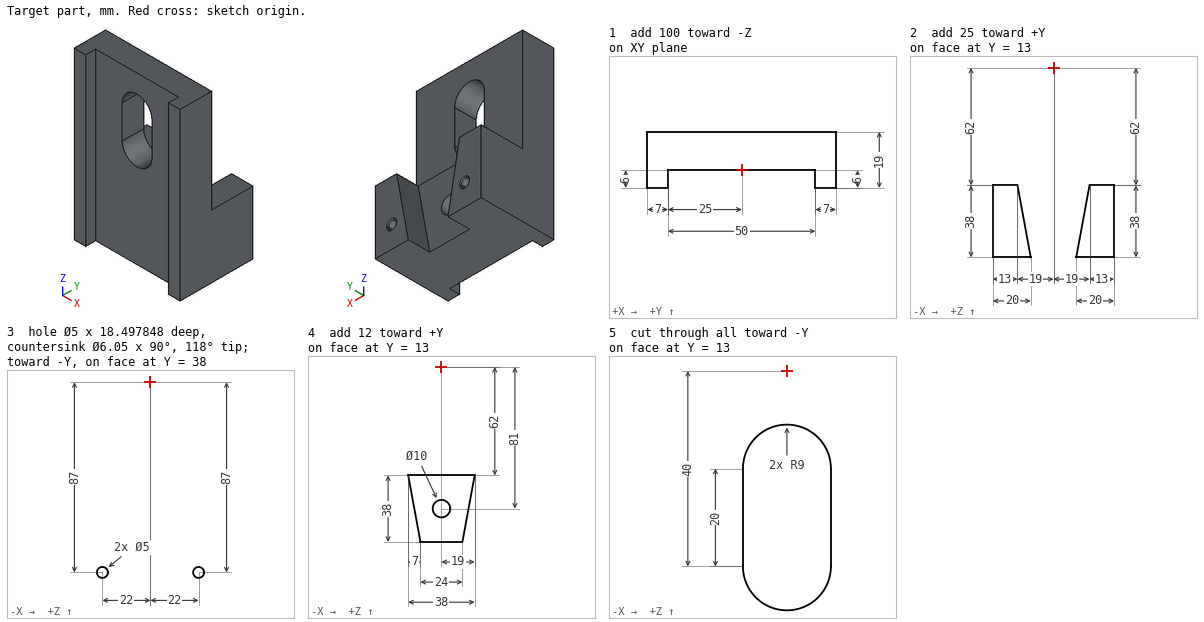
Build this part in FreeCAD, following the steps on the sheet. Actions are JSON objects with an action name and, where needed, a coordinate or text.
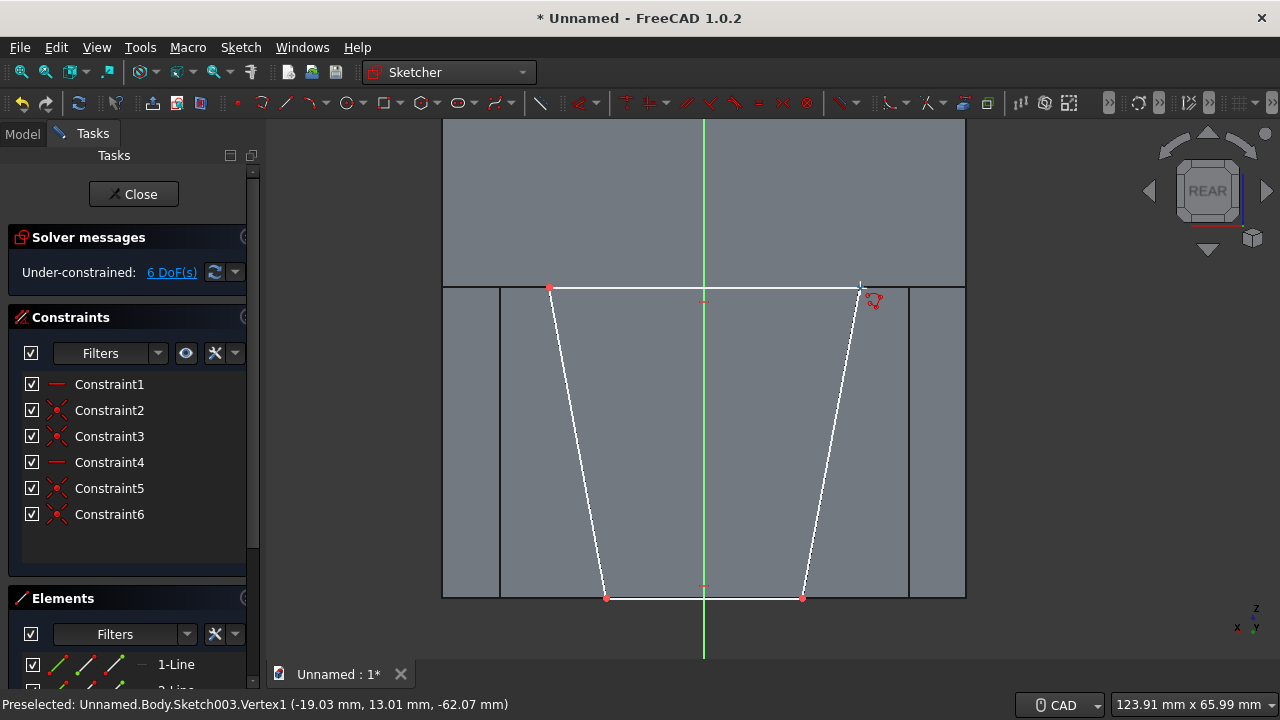
{"action": "key", "text": "g c"}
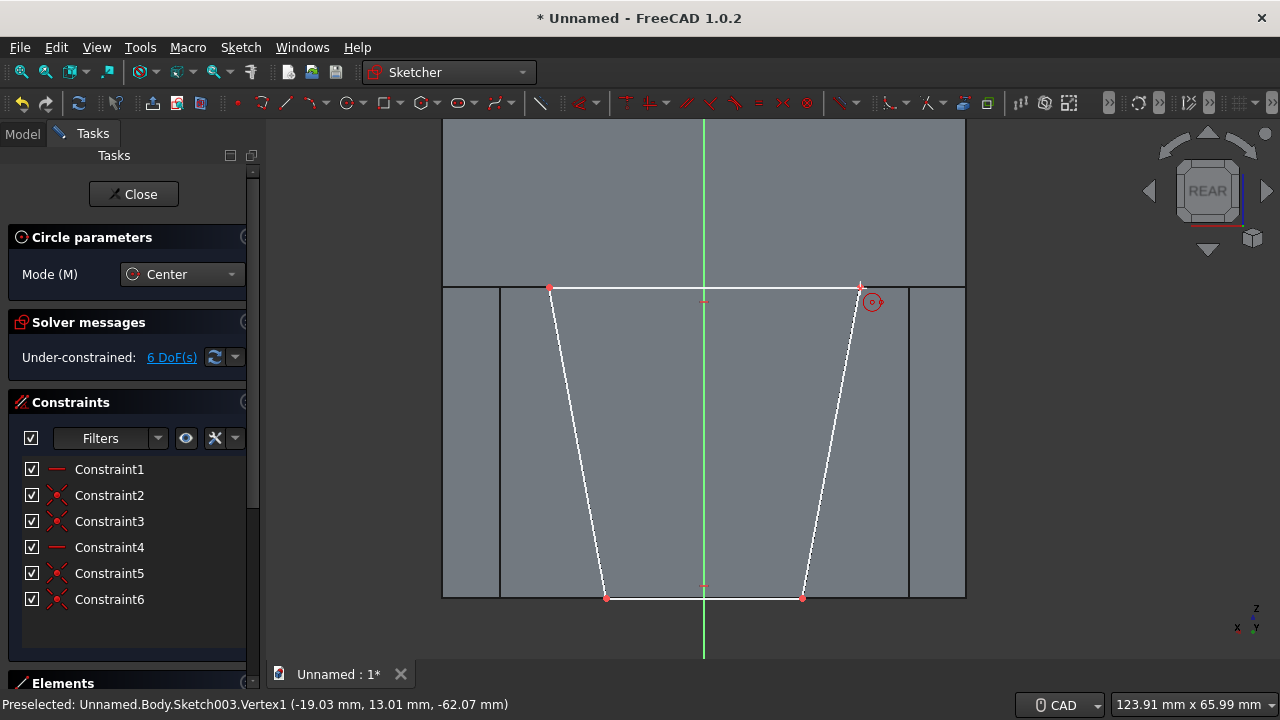
{"action": "left_click", "coordinate": [704, 443]}
{"action": "left_click", "coordinate": [733, 414]}
{"action": "key", "text": "Escape"}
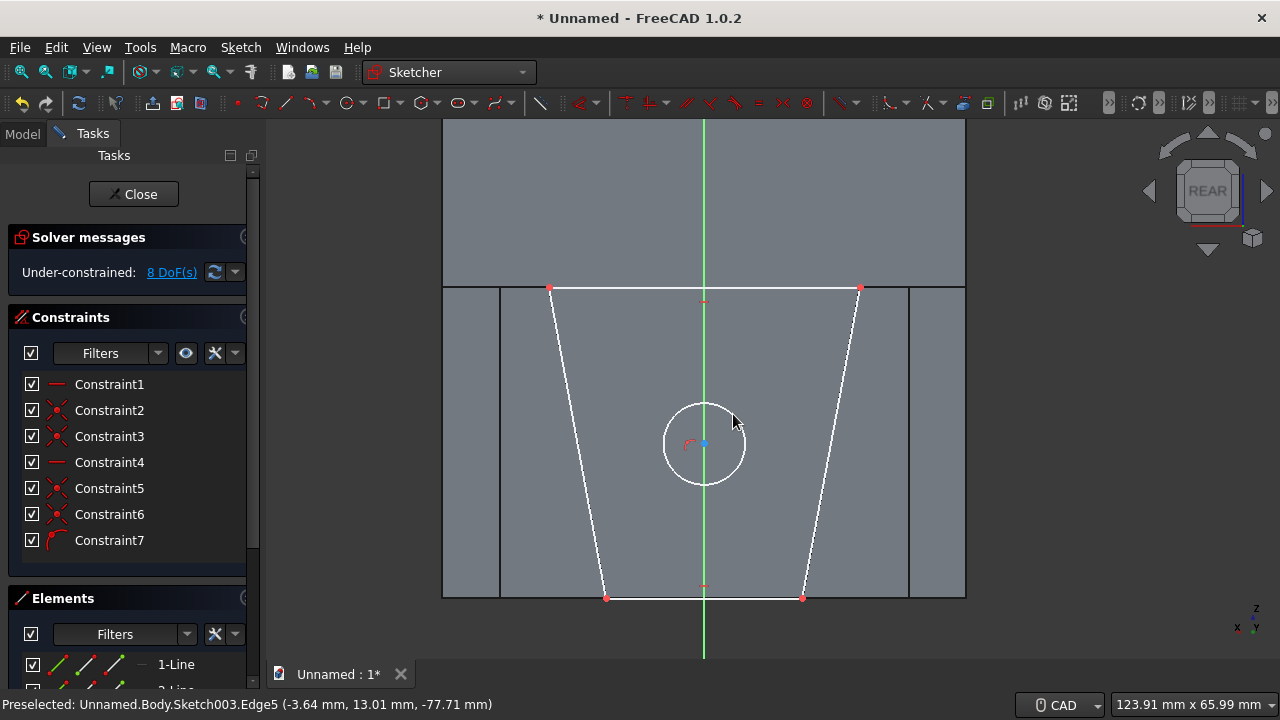
{"action": "key", "text": "d"}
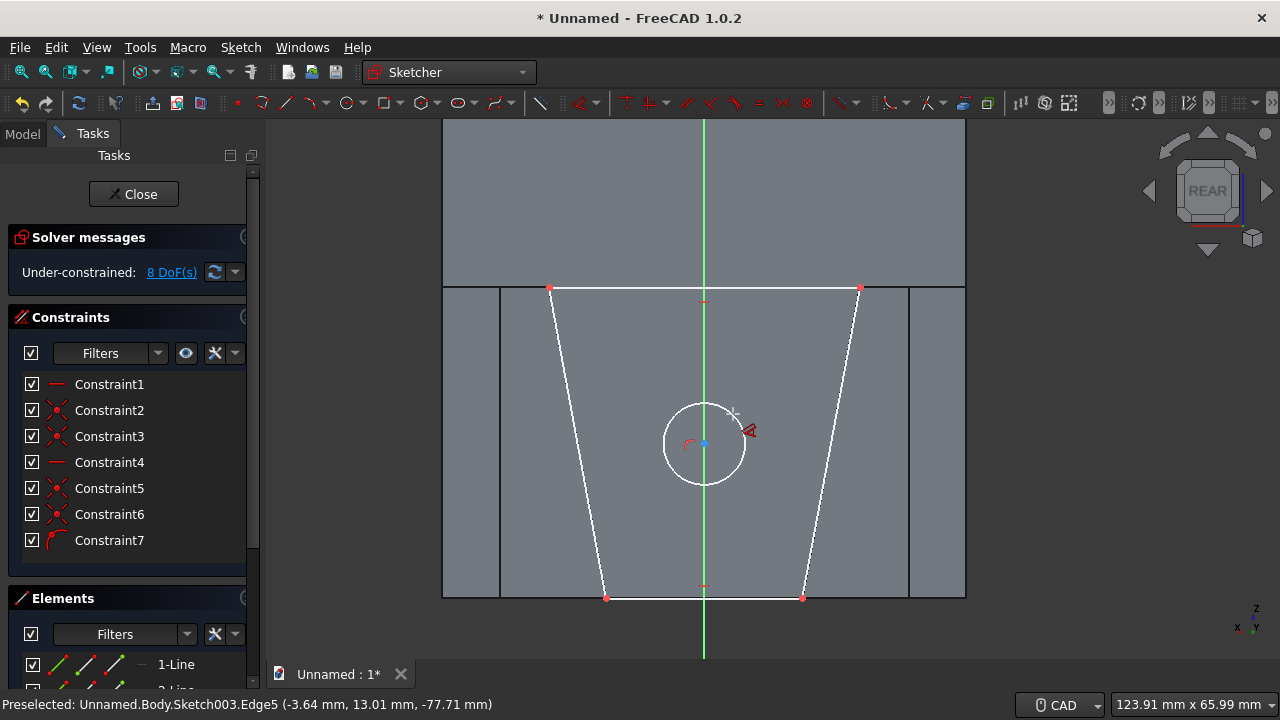
{"action": "left_click", "coordinate": [733, 415]}
{"action": "left_click", "coordinate": [756, 392]}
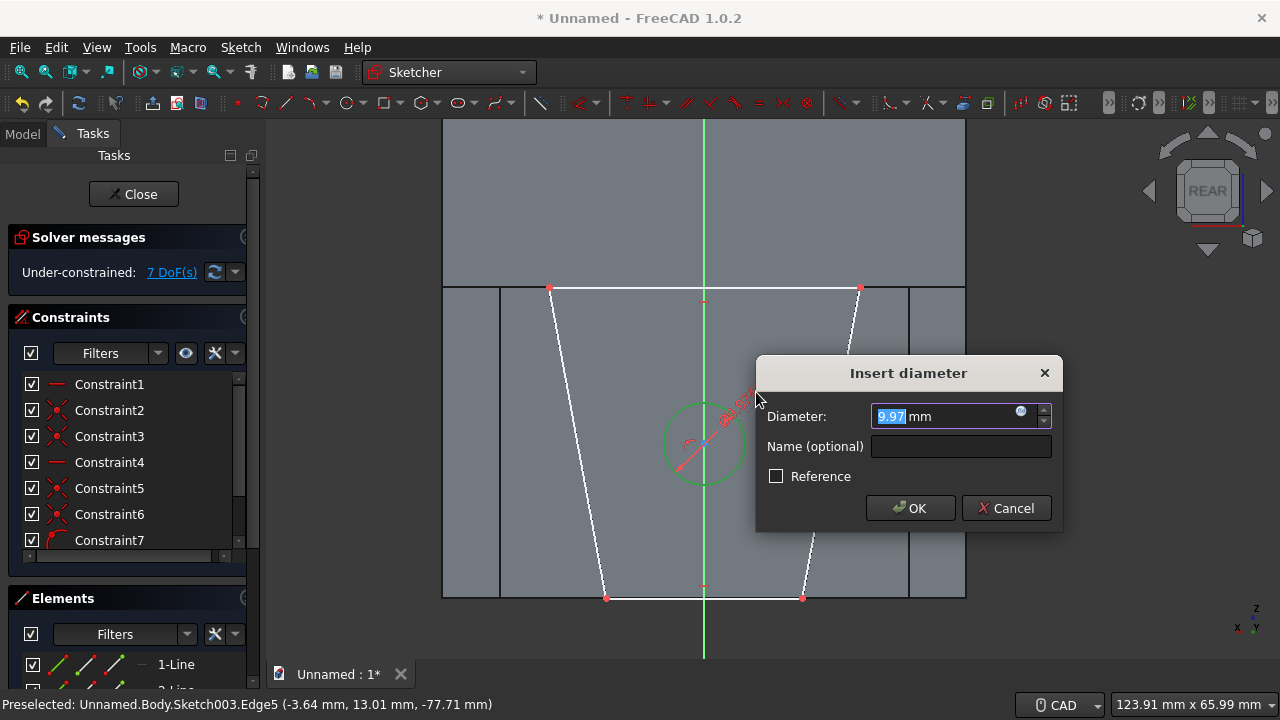
{"action": "type", "text": "10"}
{"action": "key", "text": "Return"}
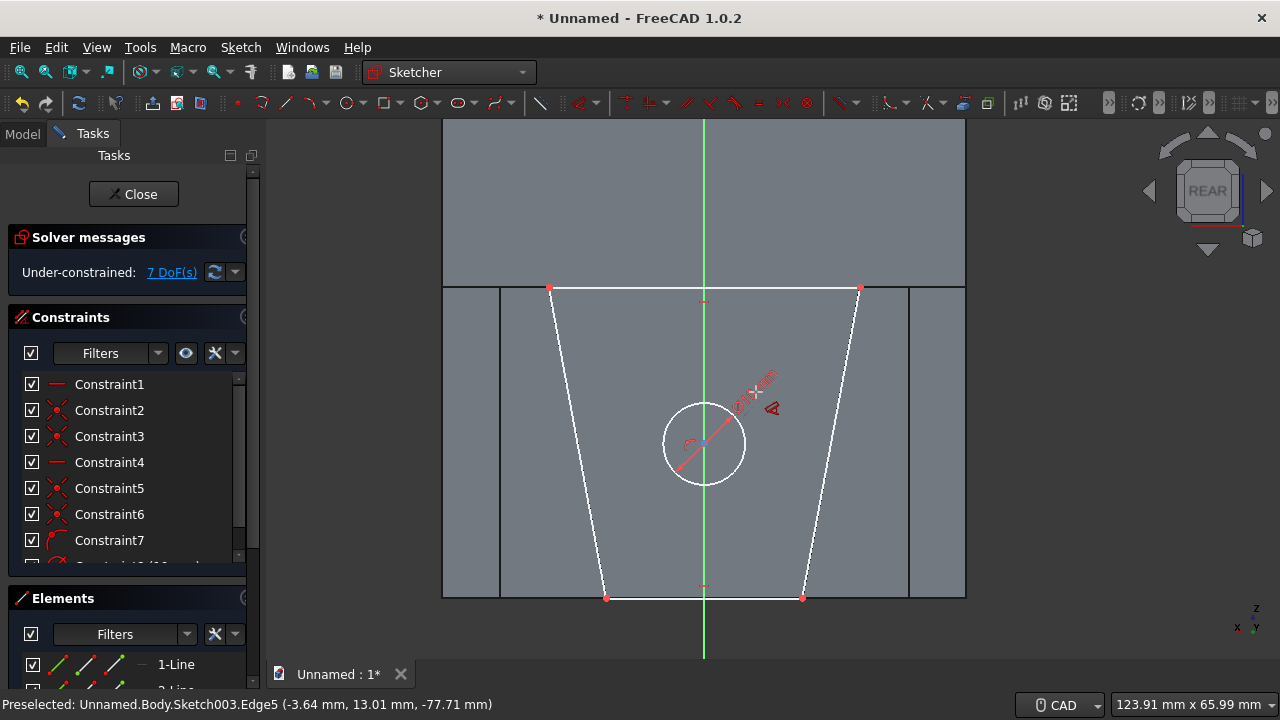
{"action": "left_click", "coordinate": [767, 288]}
{"action": "left_click", "coordinate": [633, 254]}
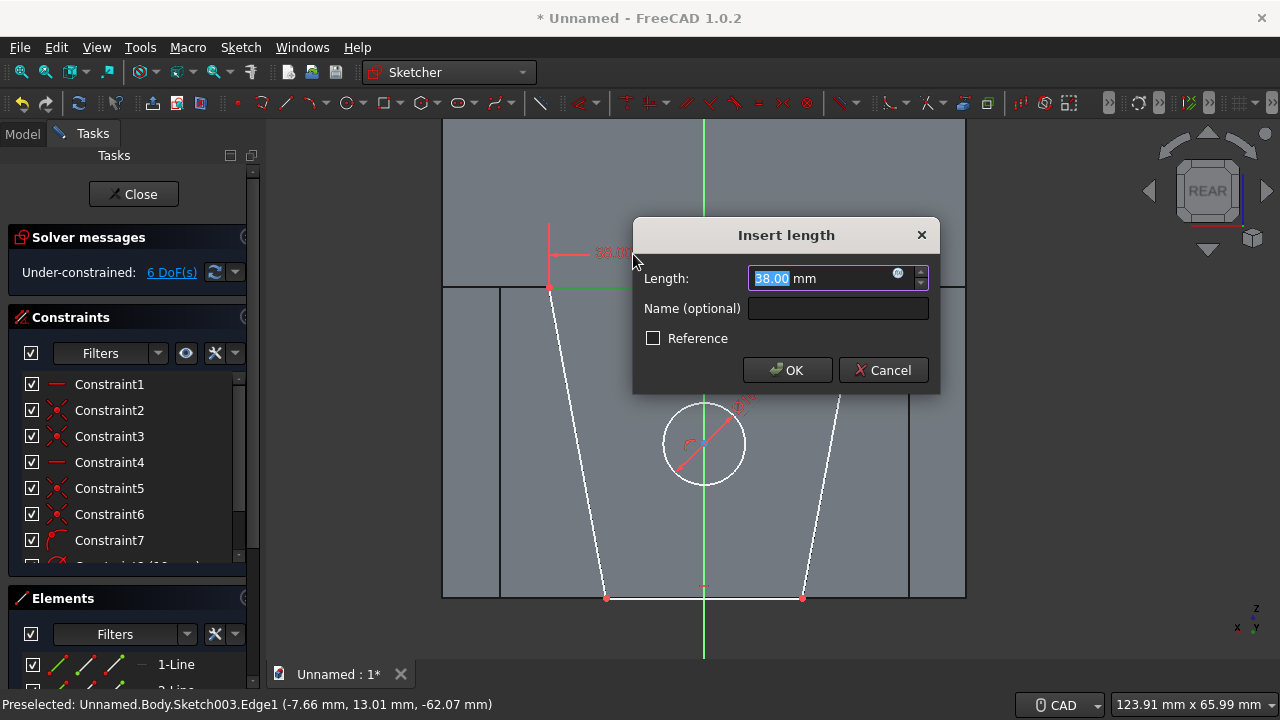
{"action": "type", "text": "38"}
{"action": "key", "text": "Return"}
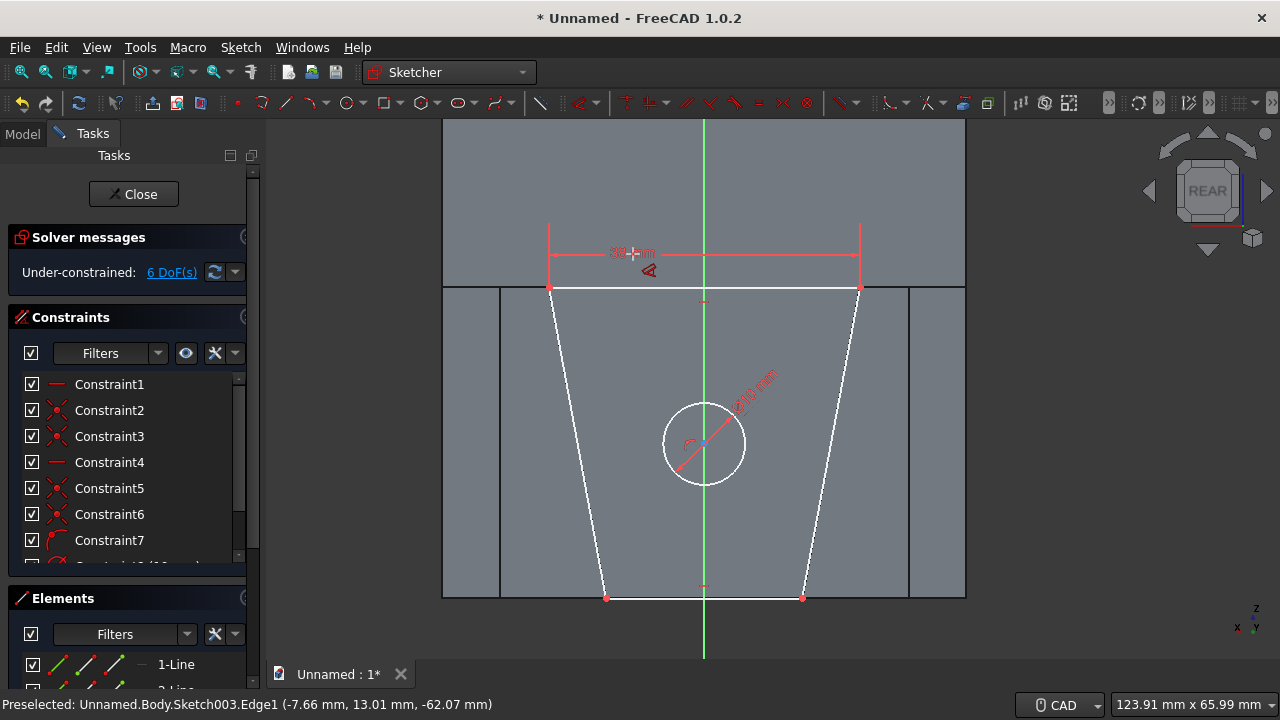
{"action": "left_click", "coordinate": [665, 599]}
{"action": "left_click", "coordinate": [659, 565]}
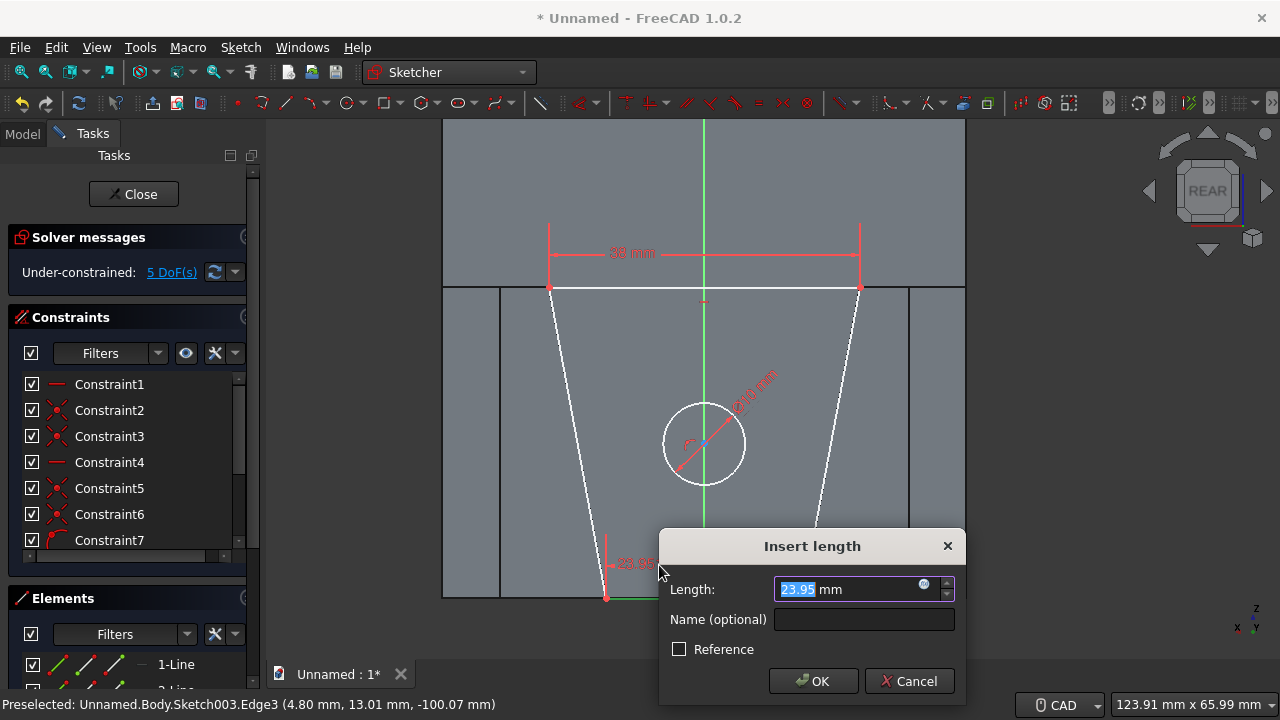
{"action": "type", "text": "24"}
{"action": "key", "text": "Return"}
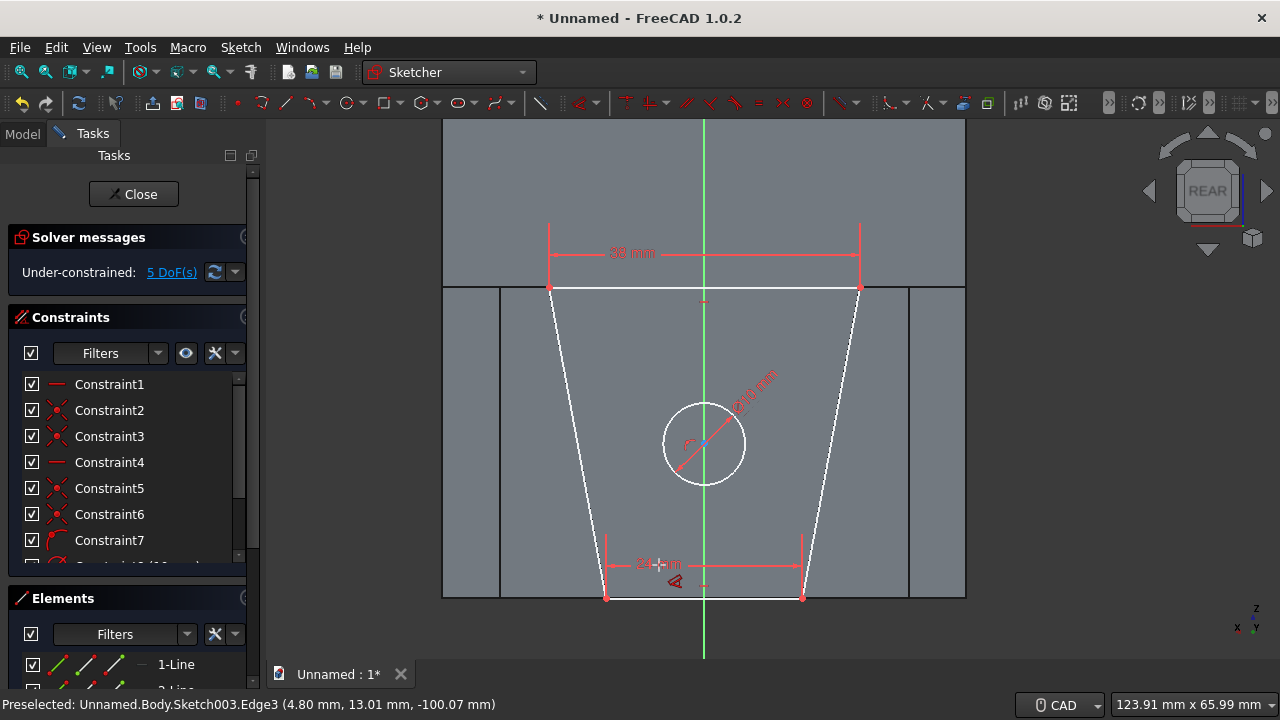
{"action": "left_click", "coordinate": [566, 381]}
{"action": "left_click", "coordinate": [558, 254]}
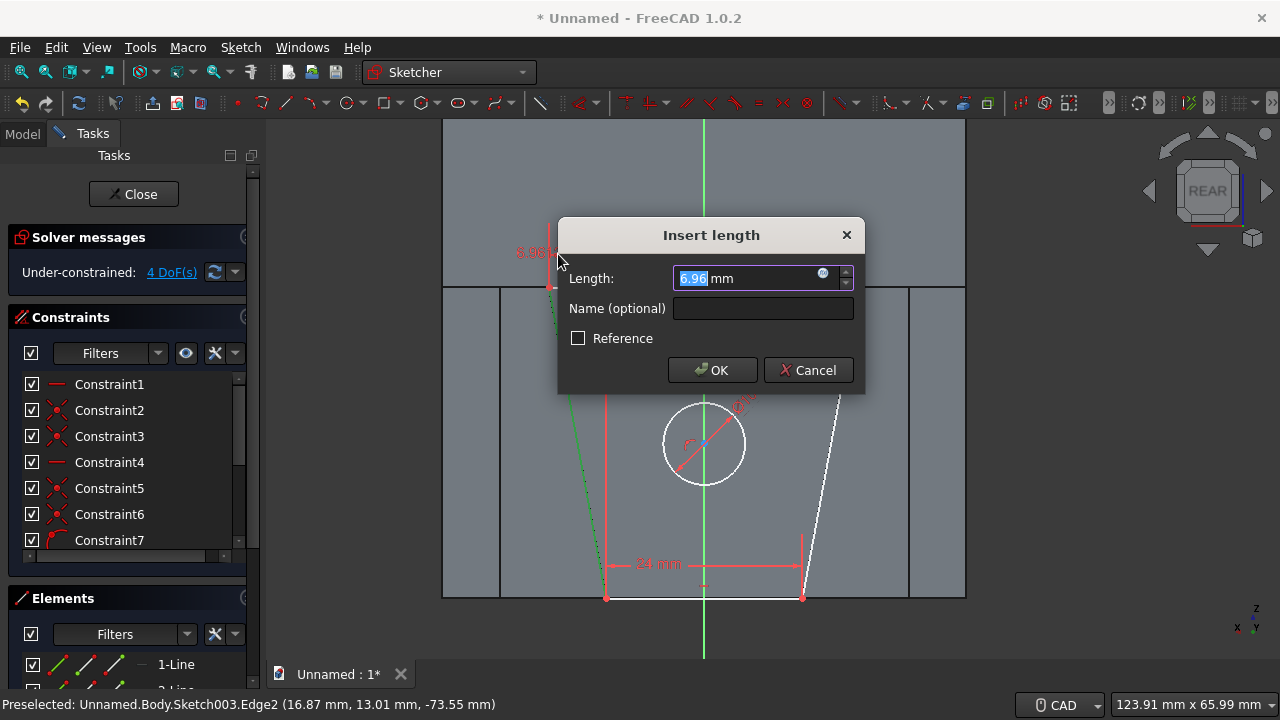
{"action": "type", "text": "7"}
{"action": "key", "text": "Return"}